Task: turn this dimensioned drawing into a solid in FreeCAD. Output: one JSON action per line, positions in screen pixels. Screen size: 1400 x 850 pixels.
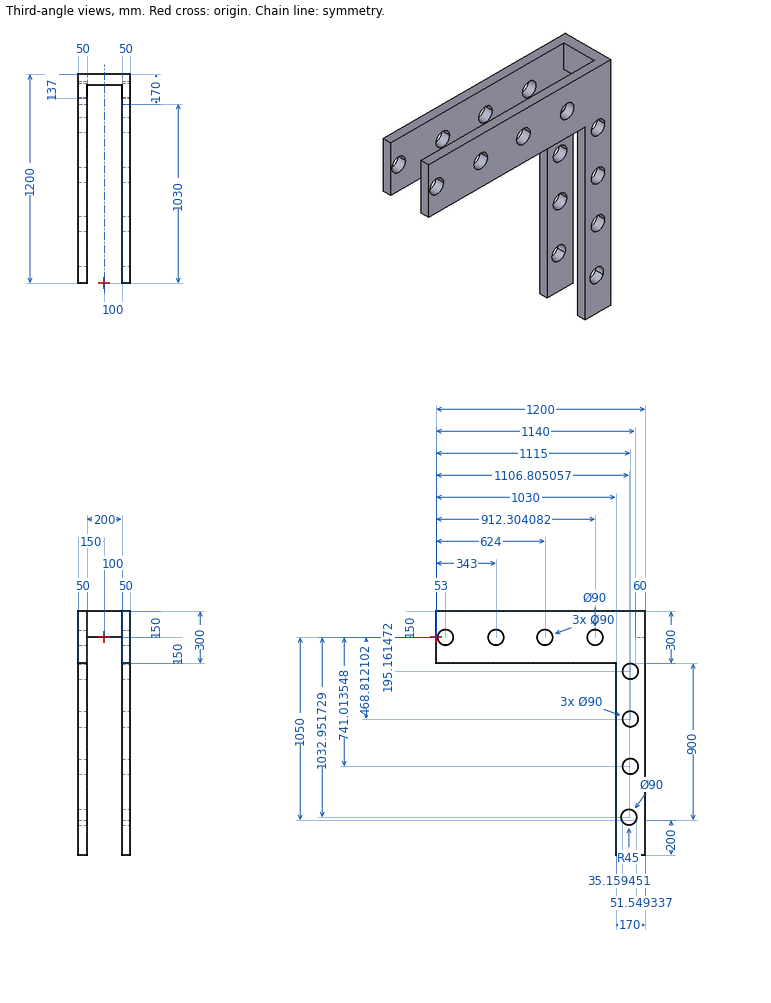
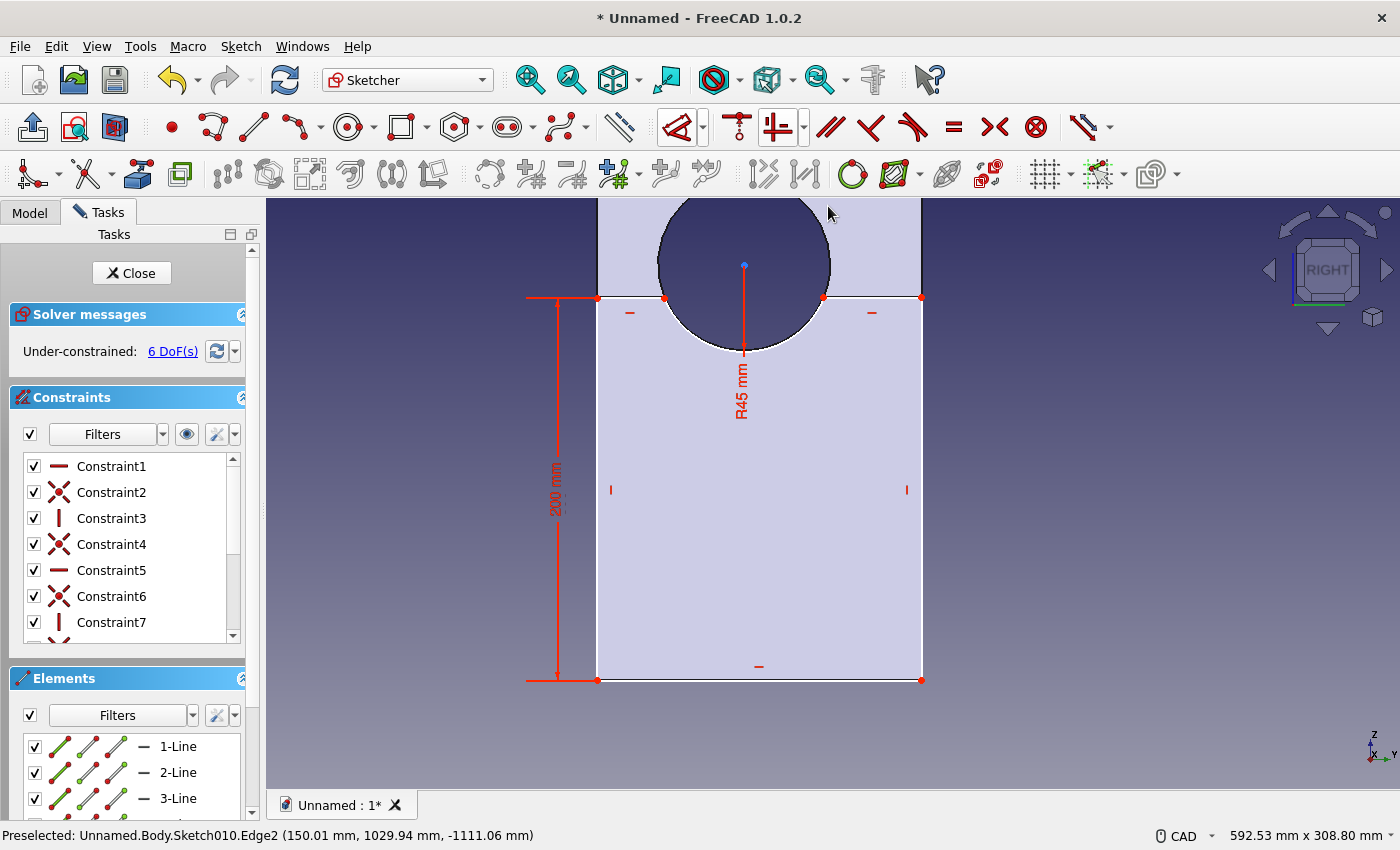
{"action": "left_click", "coordinate": [695, 681]}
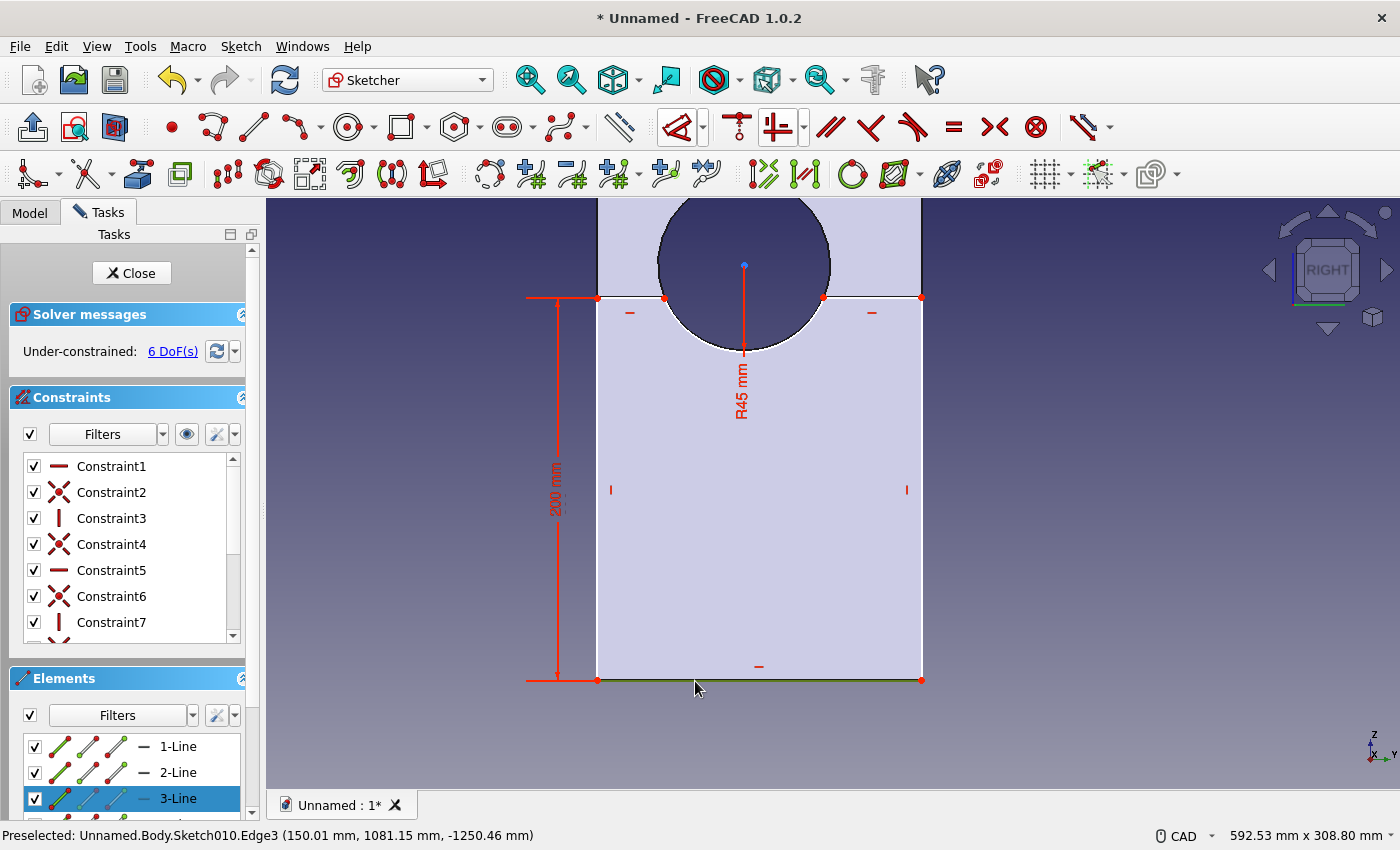
{"action": "left_click", "coordinate": [702, 128]}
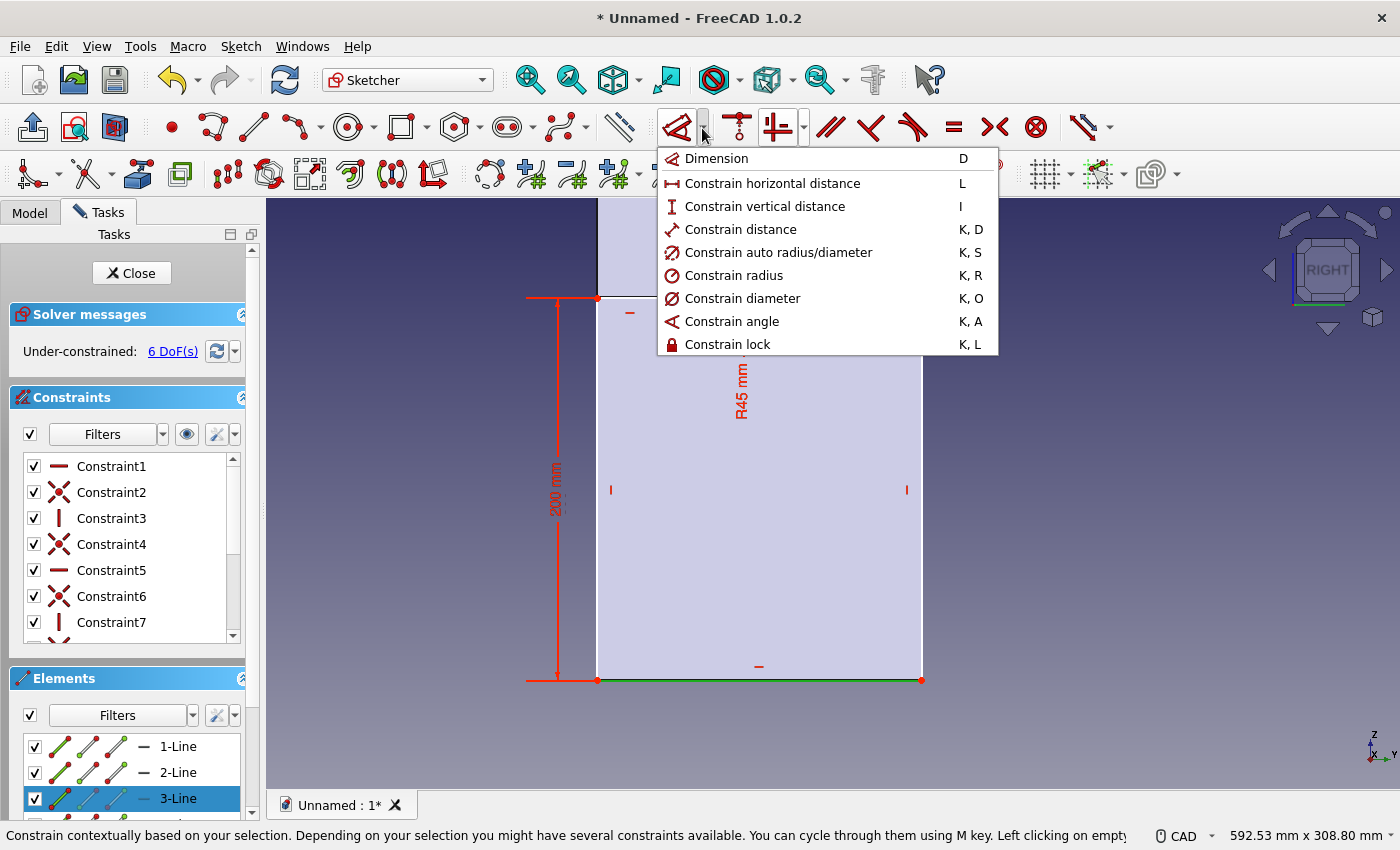
{"action": "left_click", "coordinate": [828, 184]}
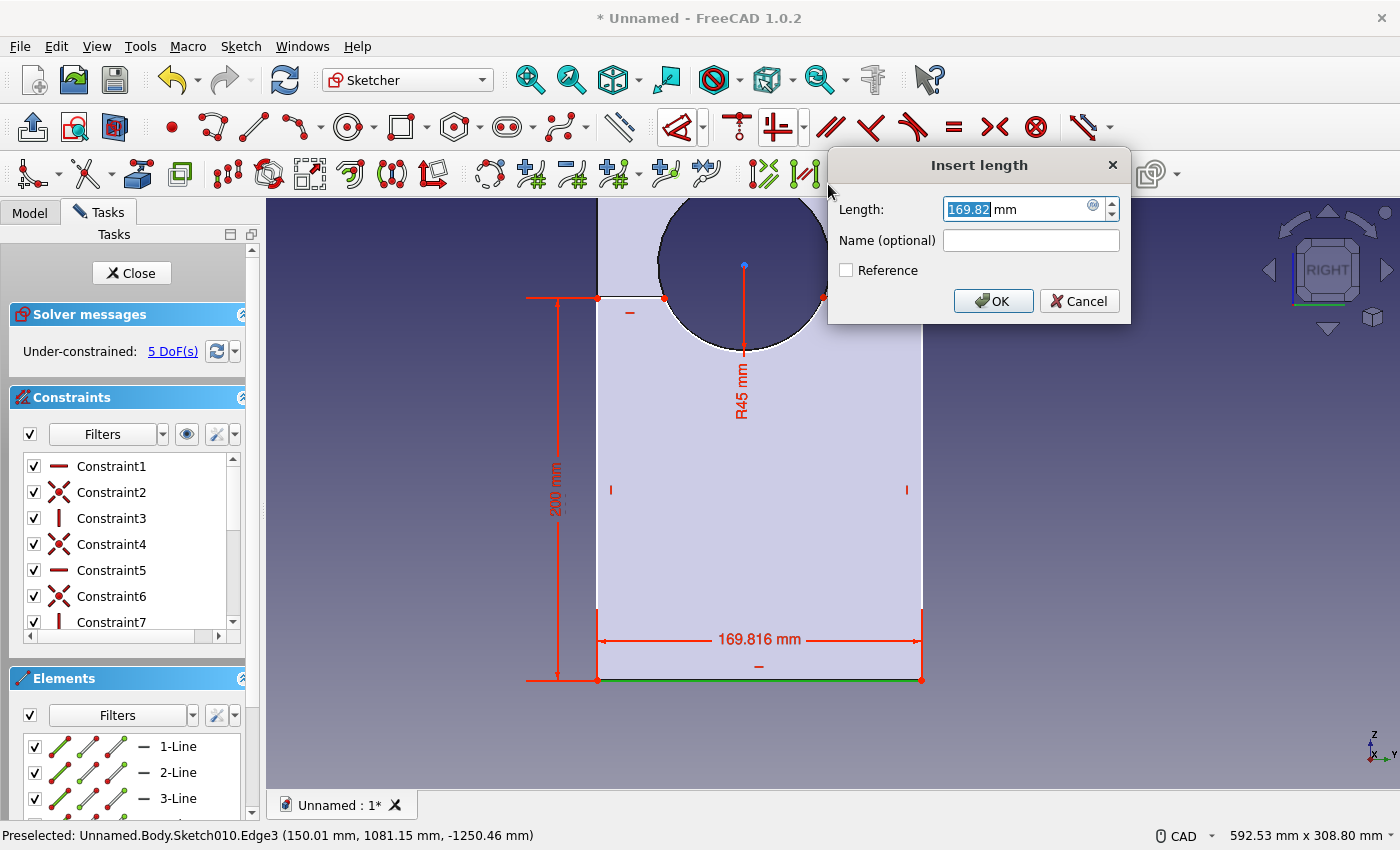
{"action": "type", "text": "170"}
{"action": "key", "text": "Return"}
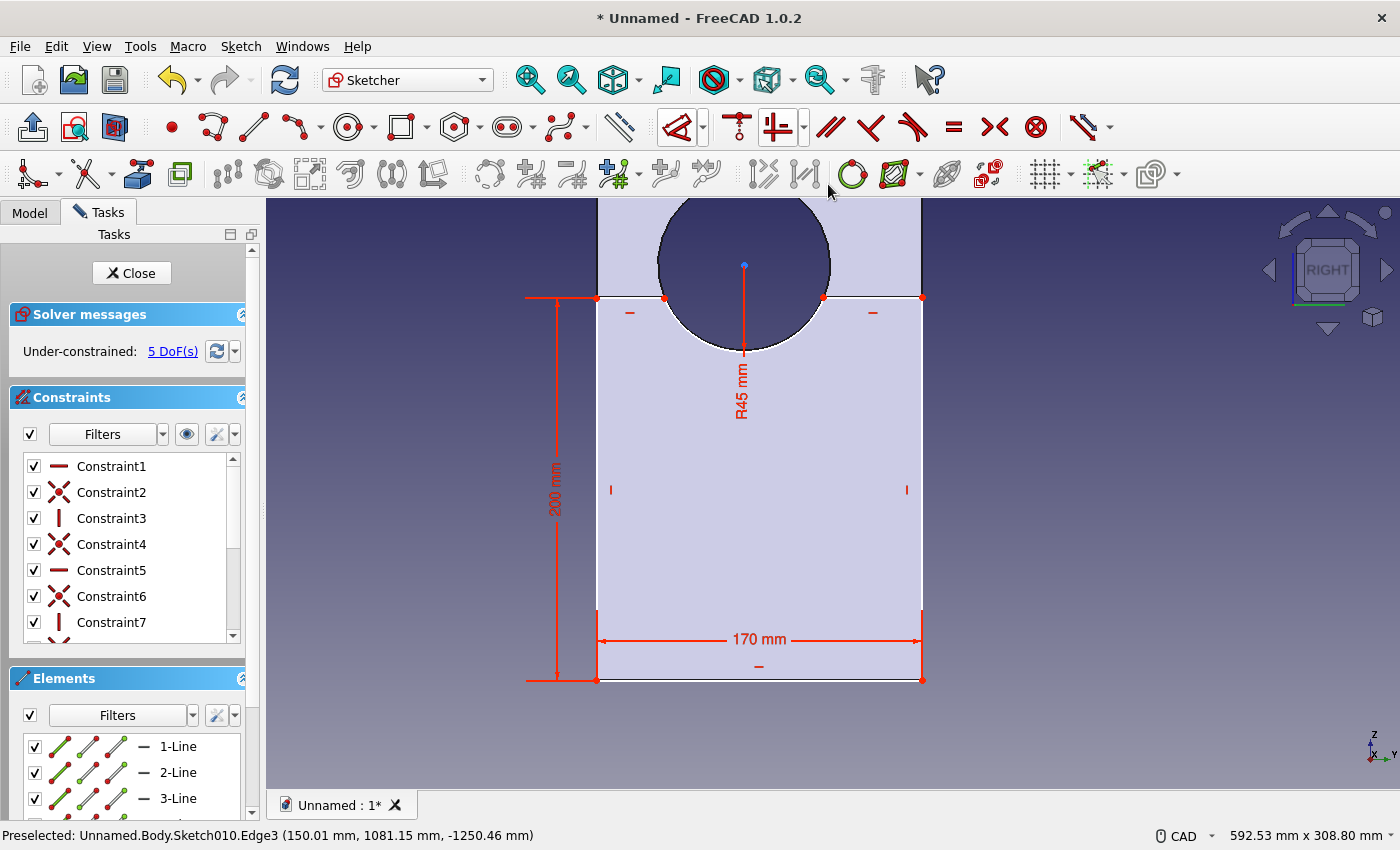
{"action": "left_click", "coordinate": [922, 566]}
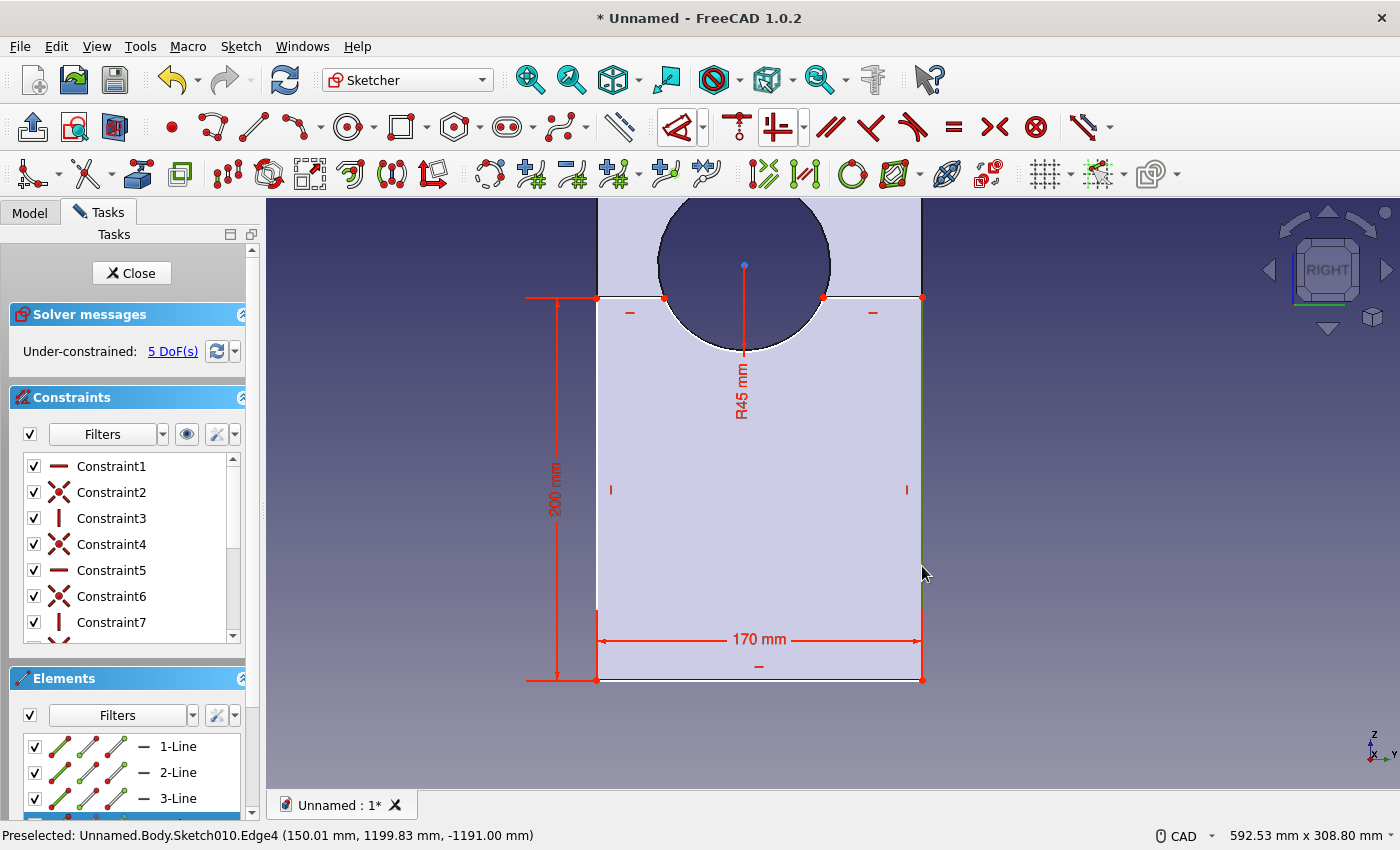
{"action": "left_click", "coordinate": [702, 128]}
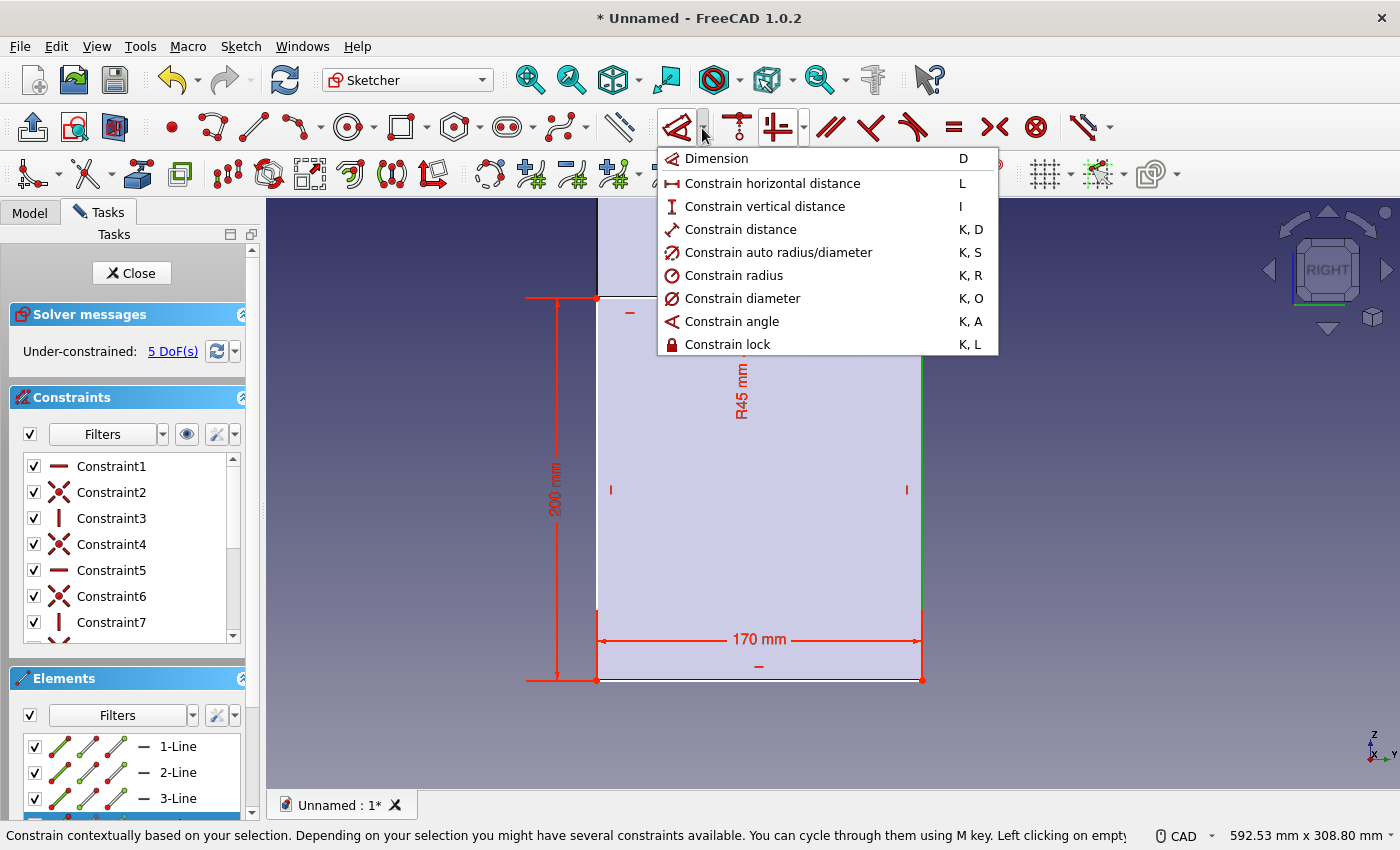
{"action": "left_click", "coordinate": [828, 206]}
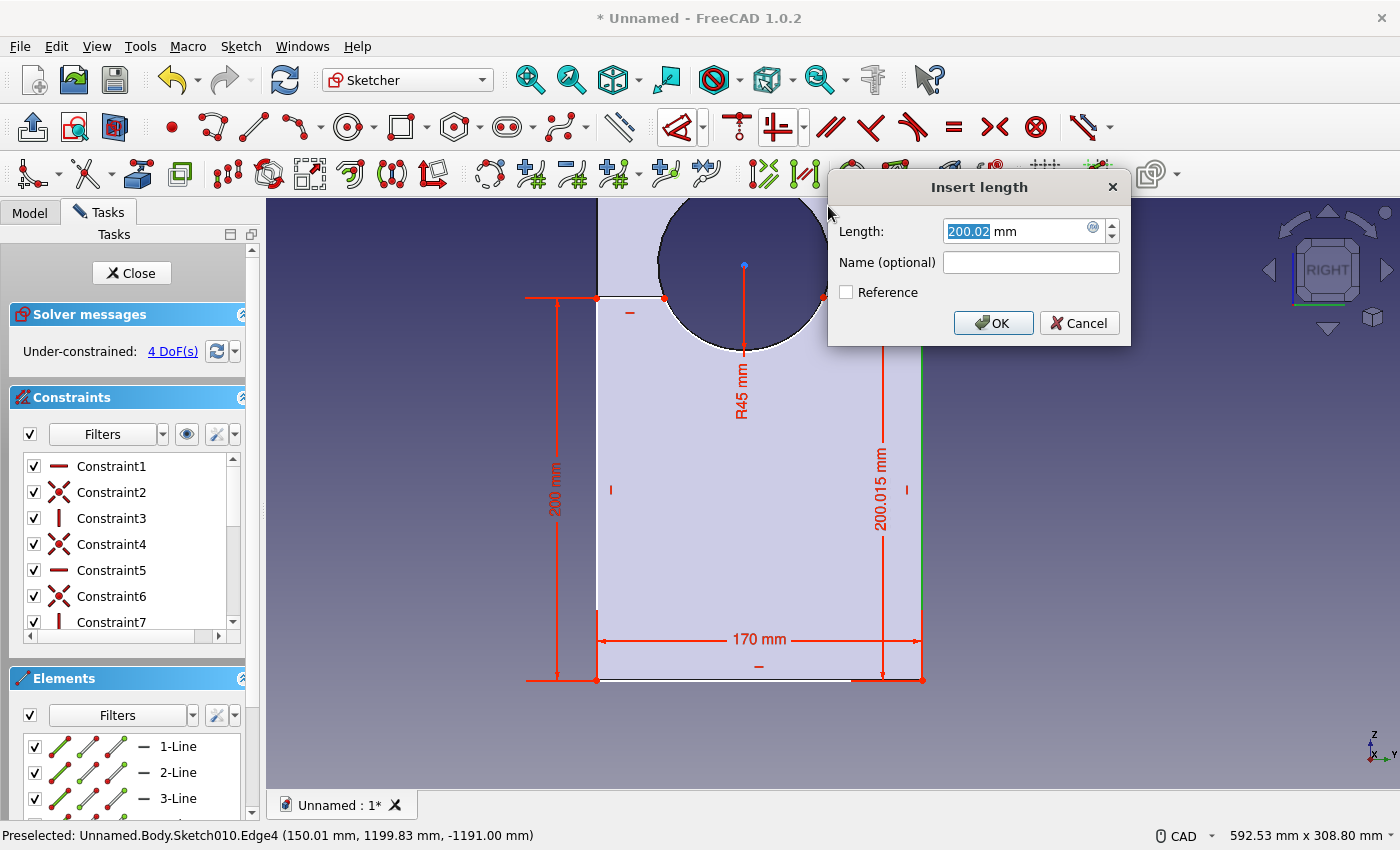
{"action": "type", "text": "200"}
{"action": "key", "text": "Return"}